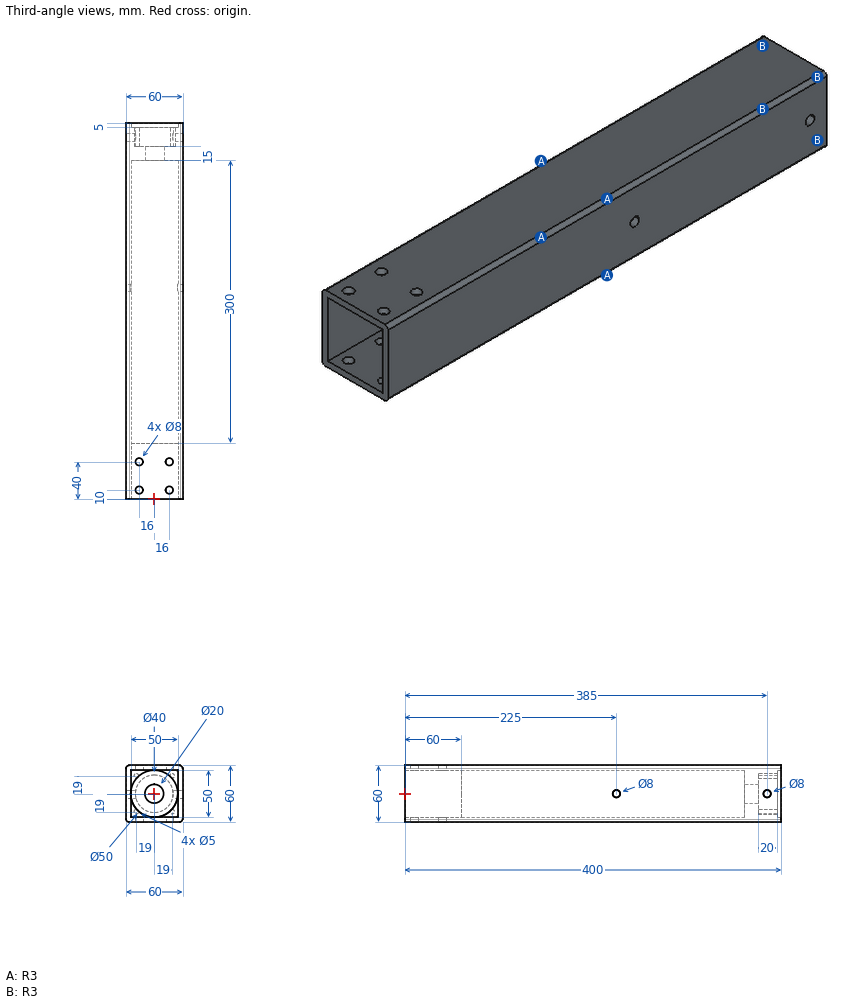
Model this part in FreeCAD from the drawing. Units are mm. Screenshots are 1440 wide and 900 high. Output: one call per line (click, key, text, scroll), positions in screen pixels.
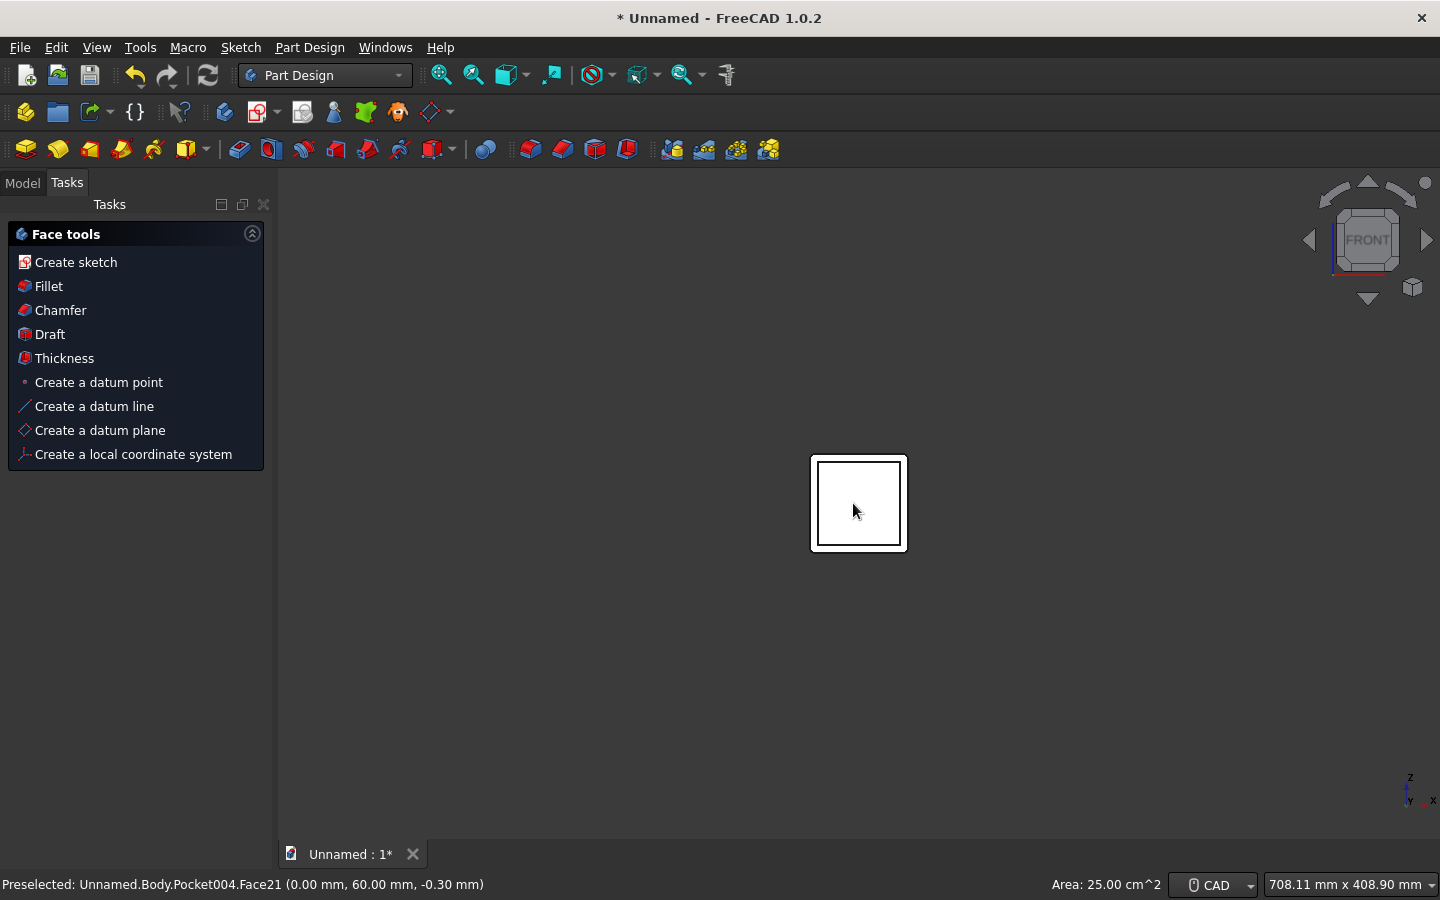
click(258, 112)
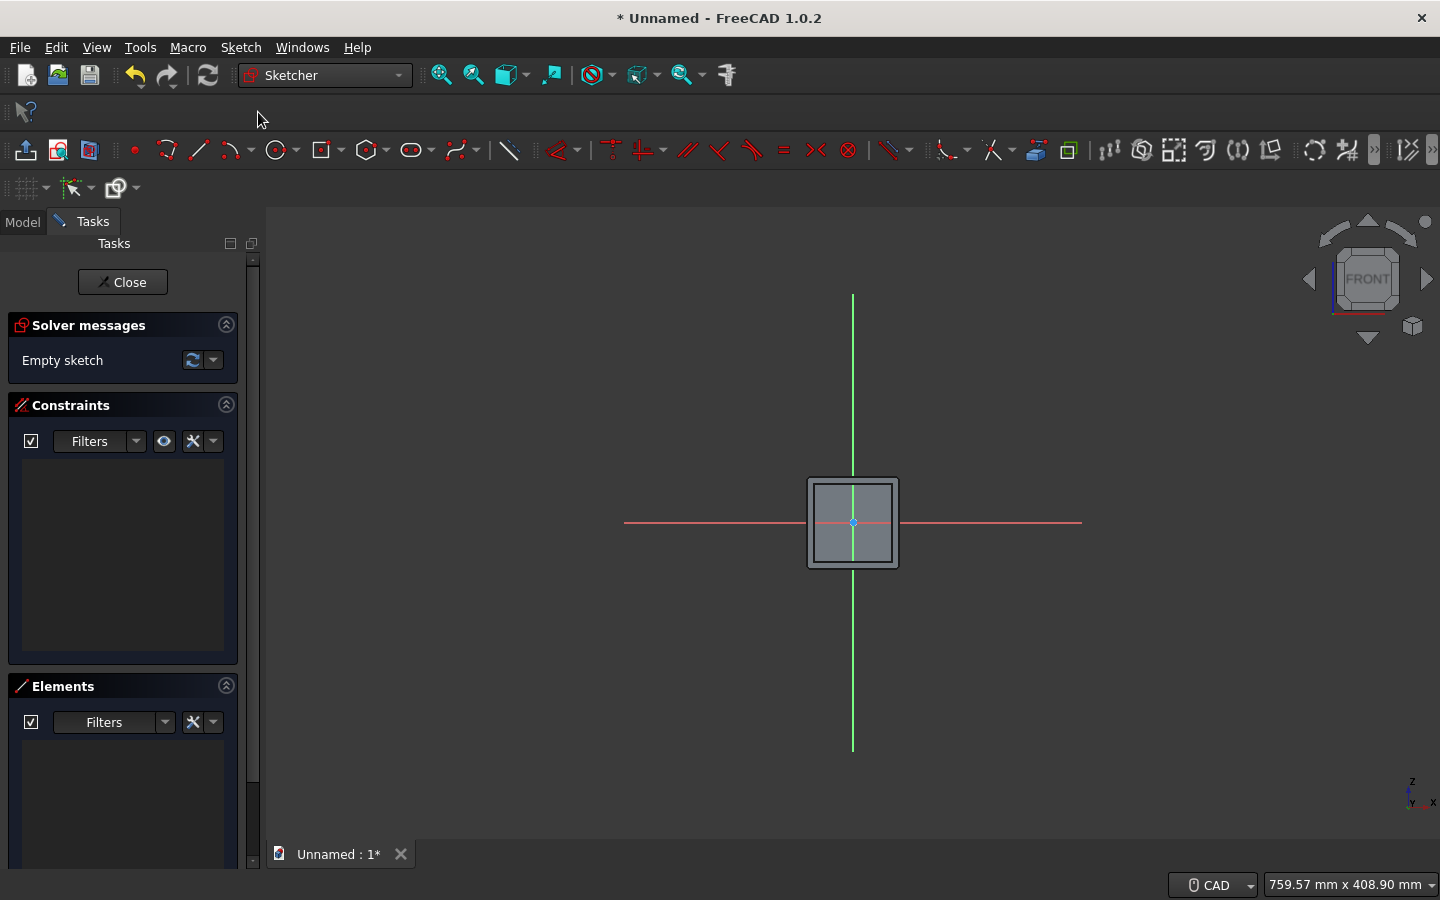
scroll(870, 523, up, 8)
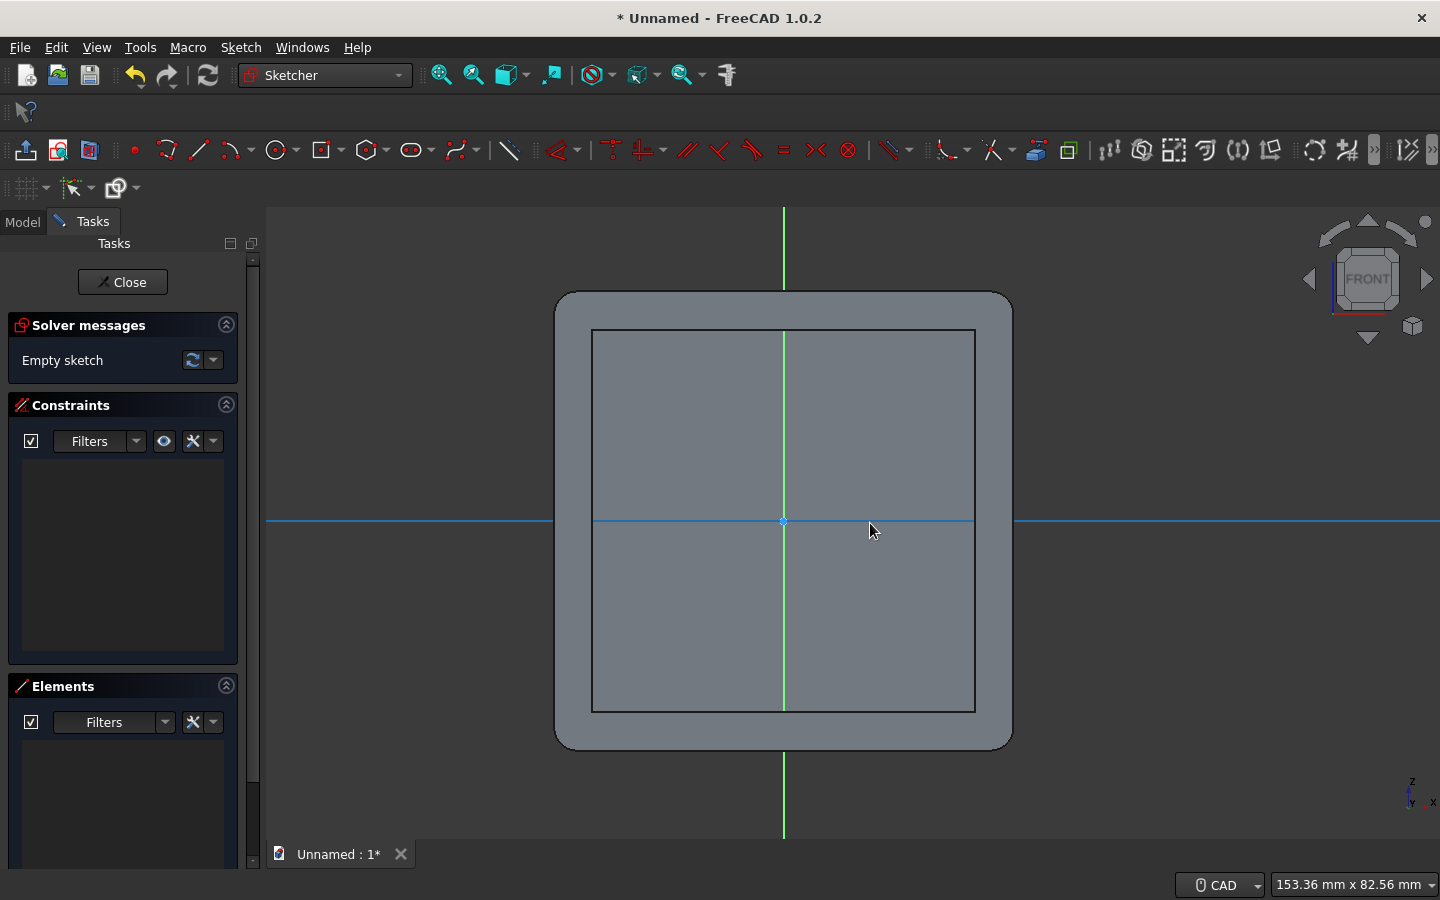
click(276, 150)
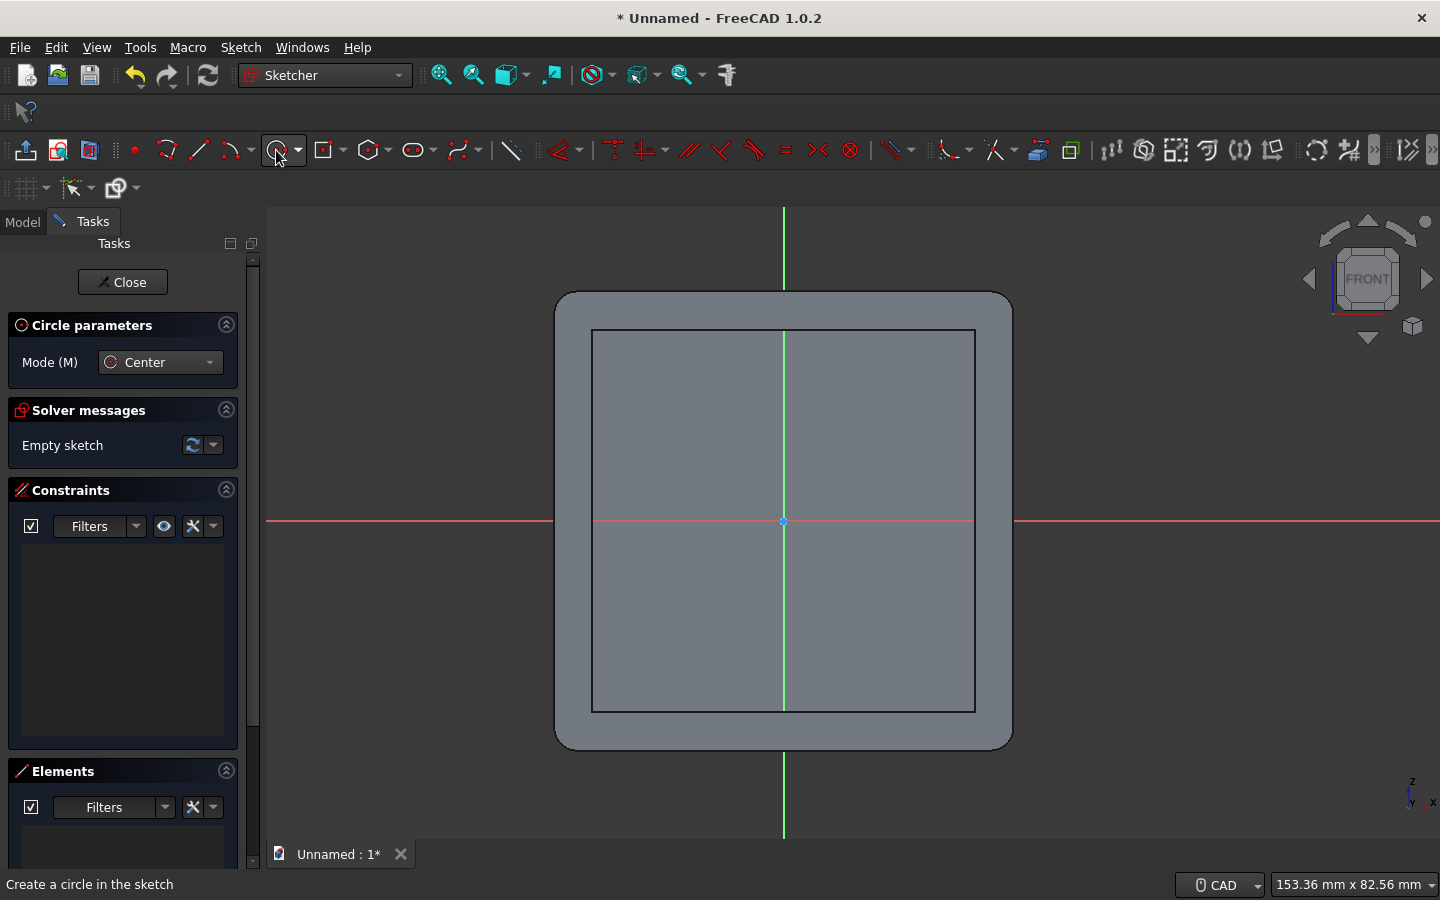
click(784, 521)
move(919, 386)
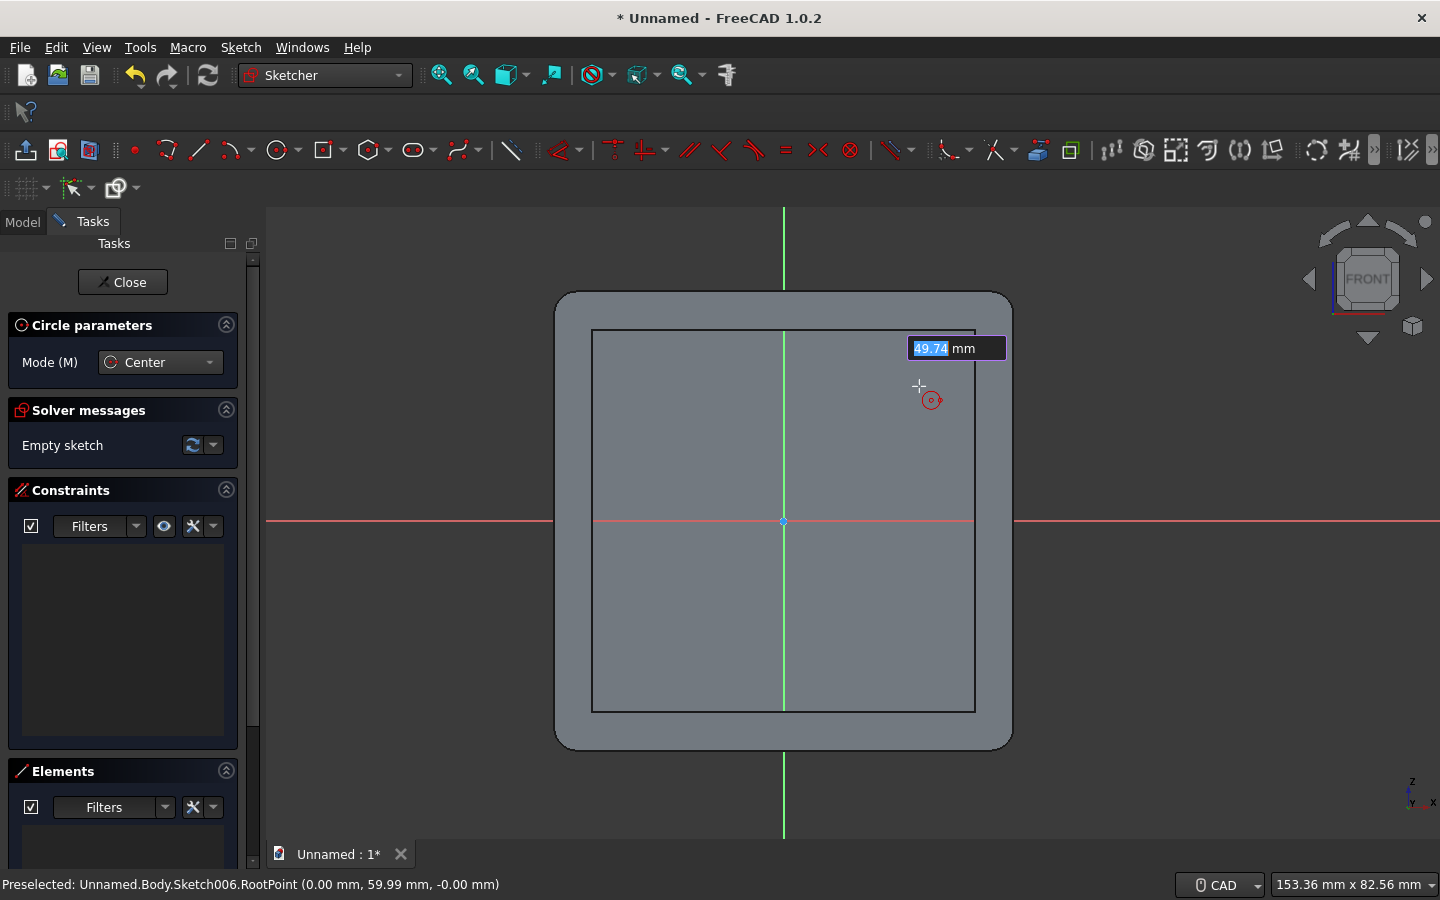
text(50)
key(Return)
key(Escape)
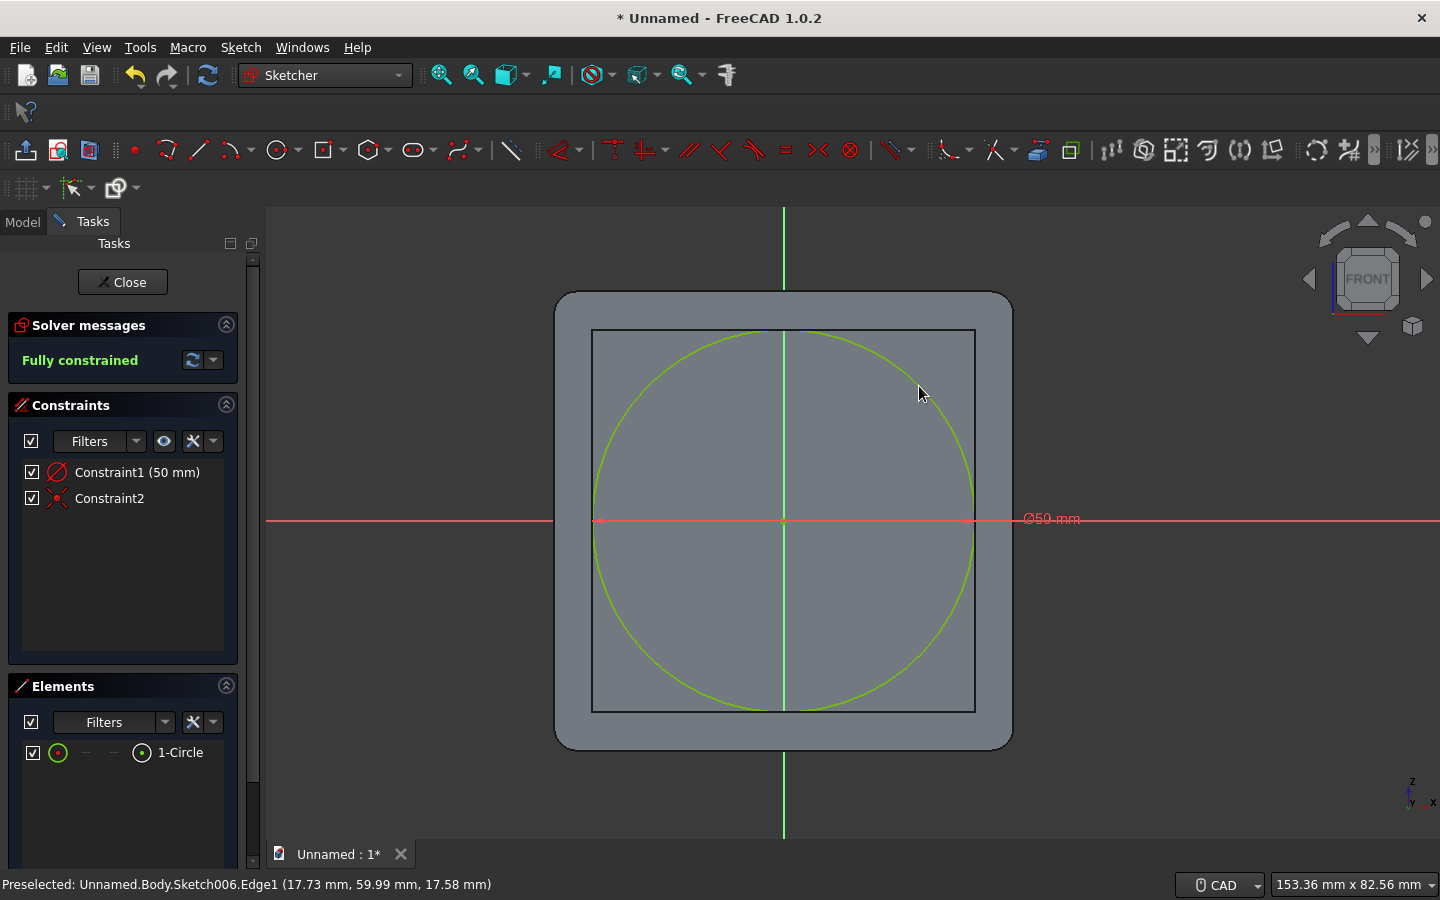
click(123, 282)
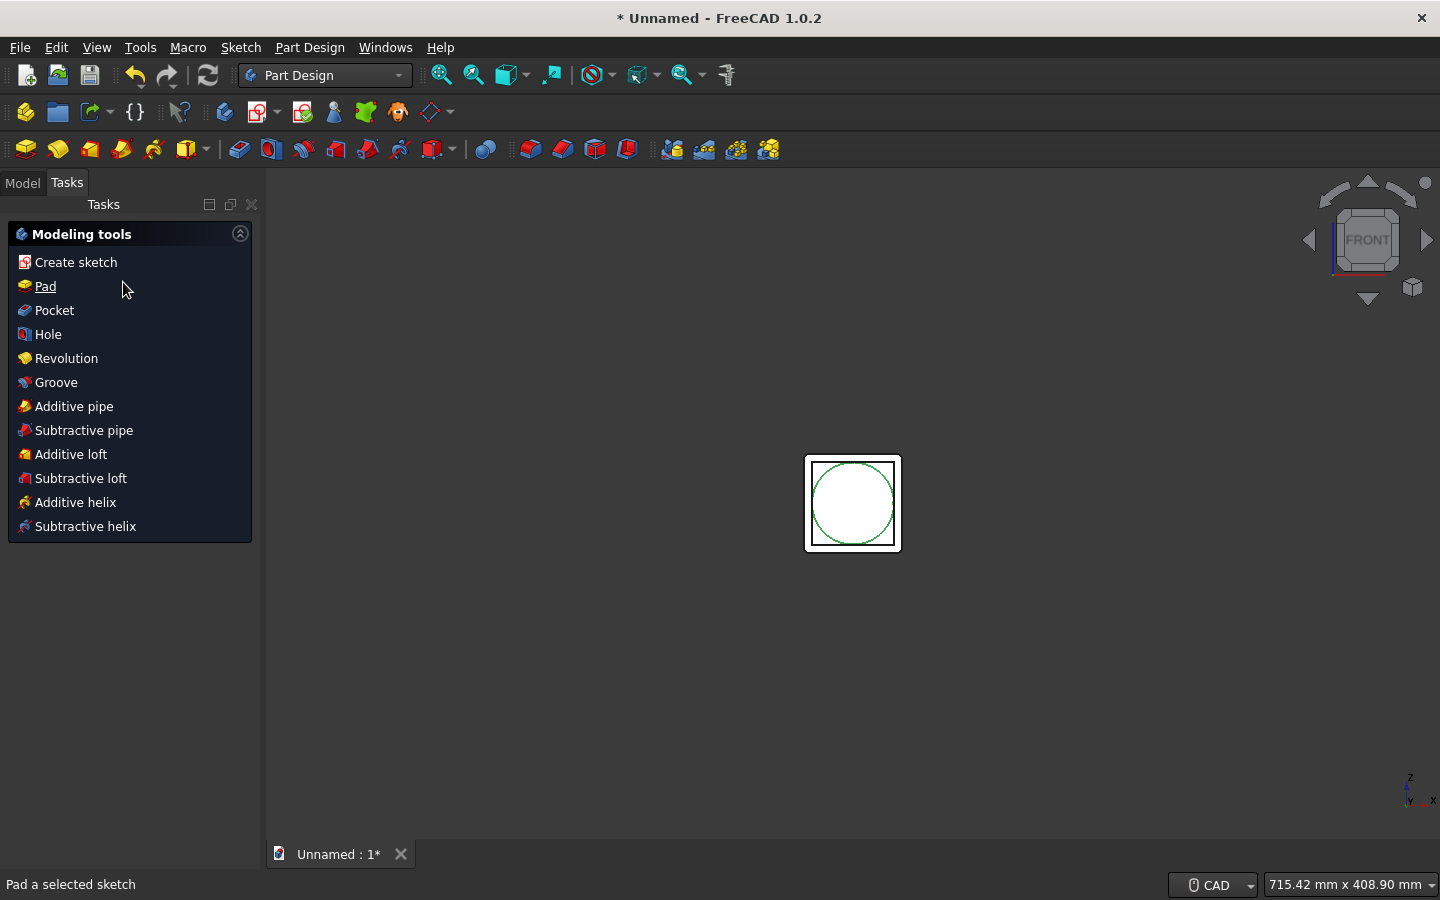
click(240, 150)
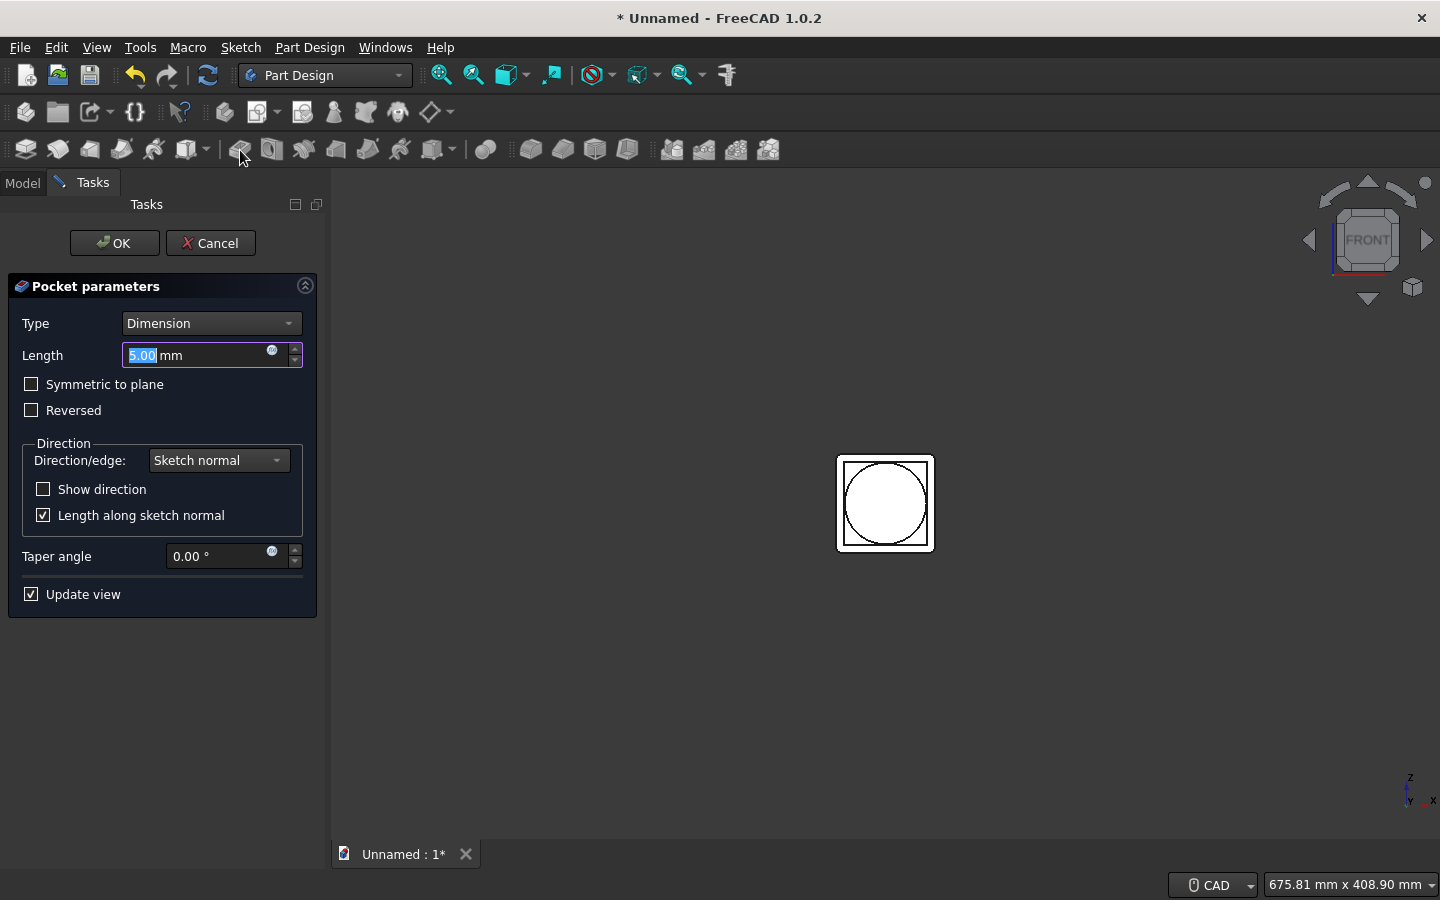
text(300)
key(Tab)